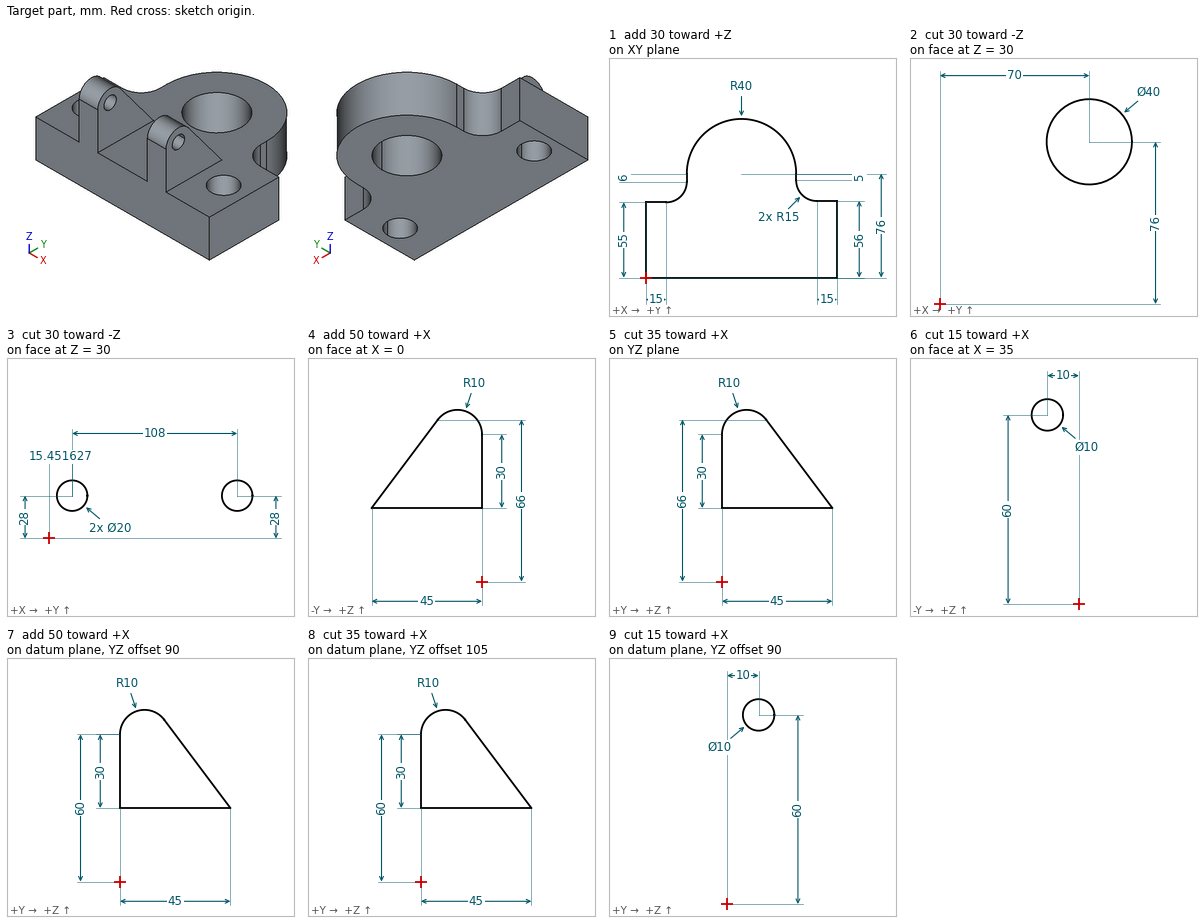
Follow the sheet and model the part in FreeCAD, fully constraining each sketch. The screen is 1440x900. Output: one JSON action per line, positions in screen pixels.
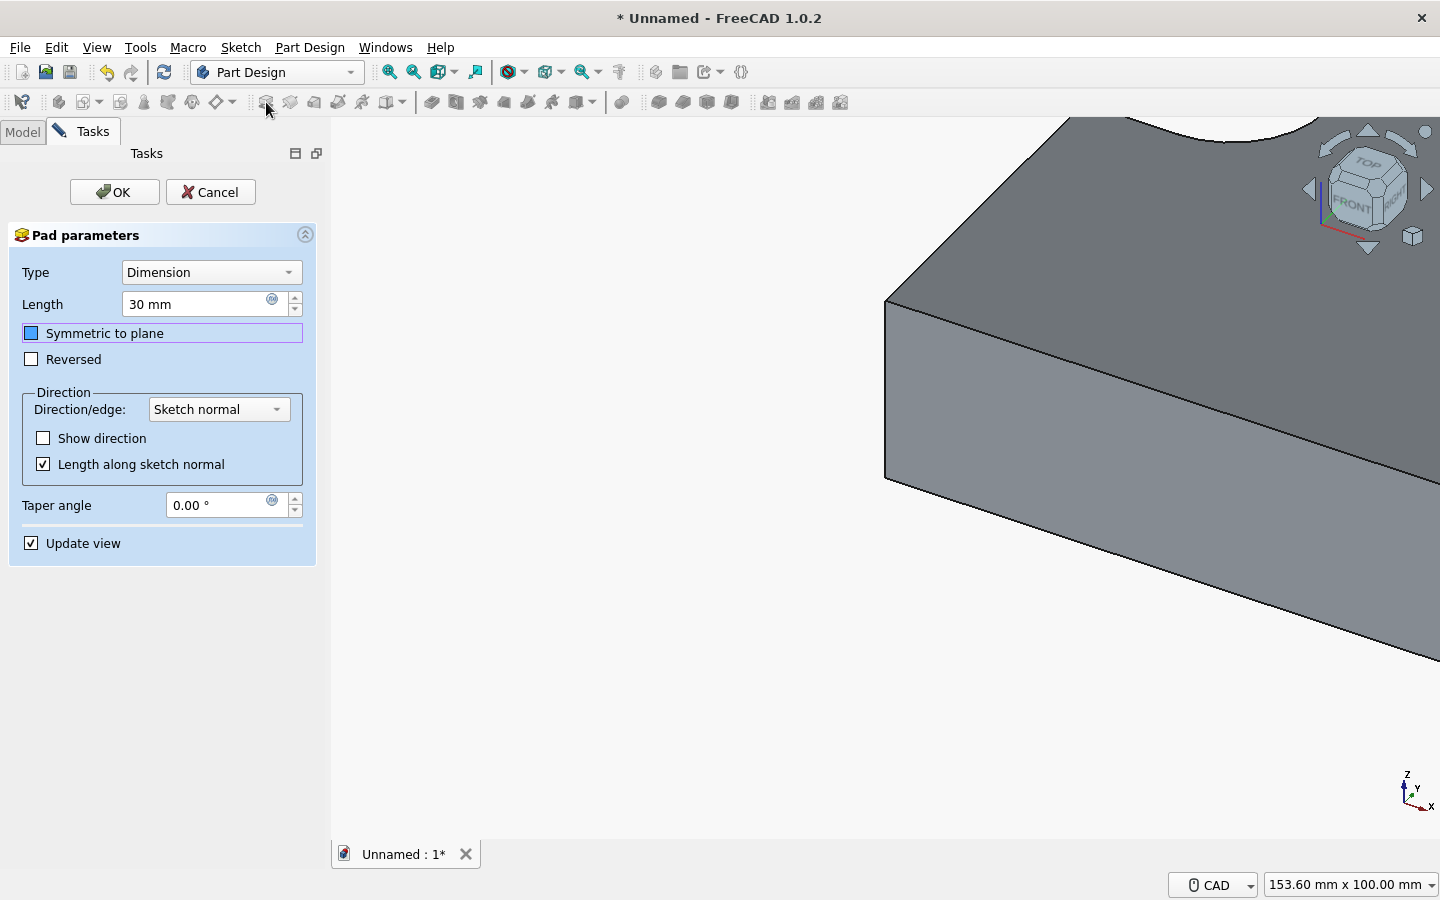
{"action": "left_click", "coordinate": [115, 192]}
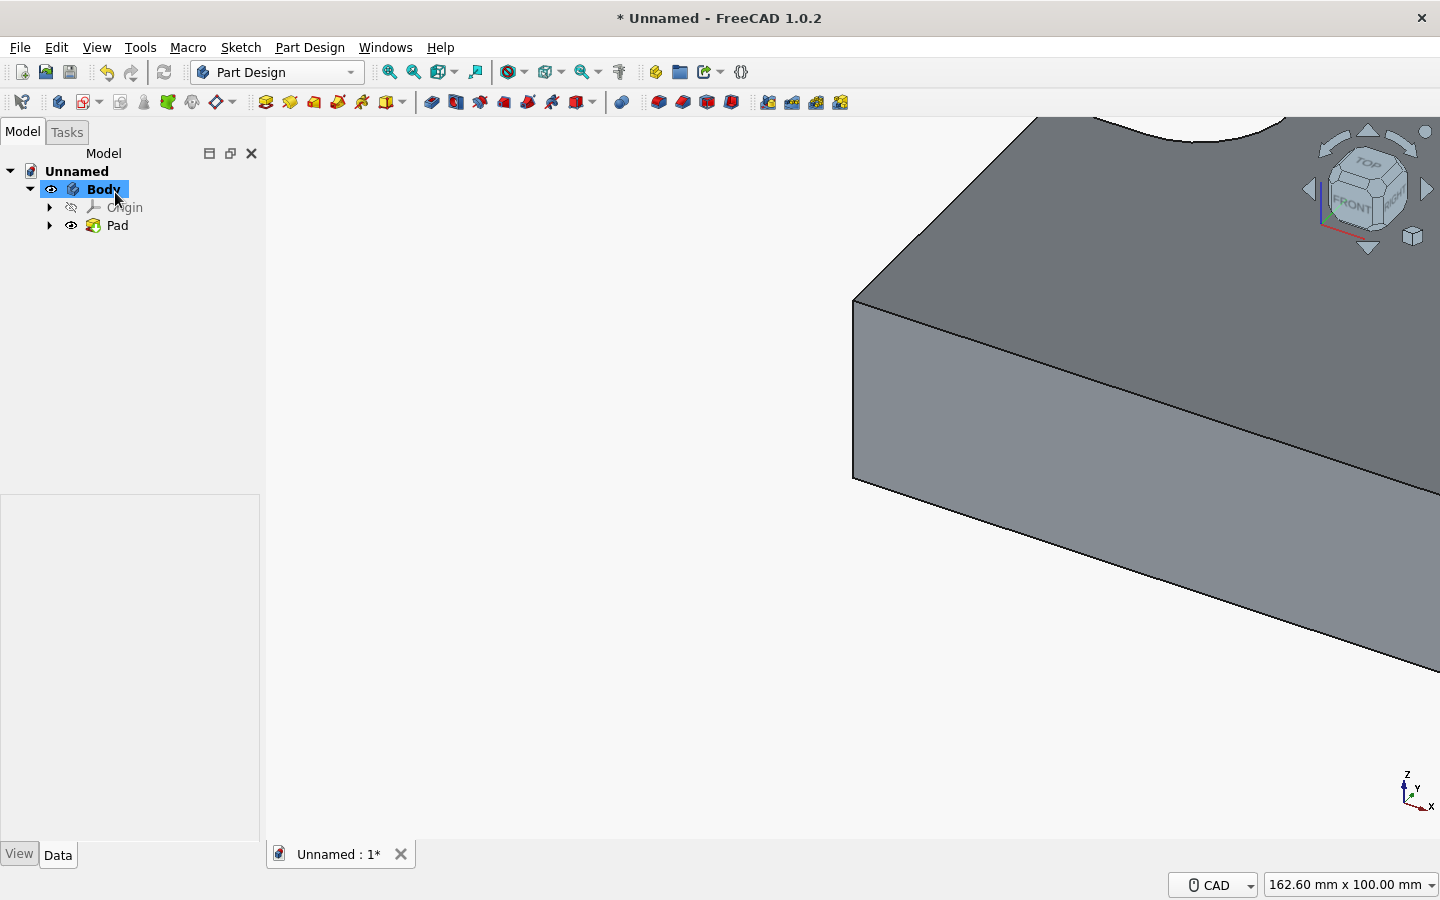
{"action": "key", "text": "v f"}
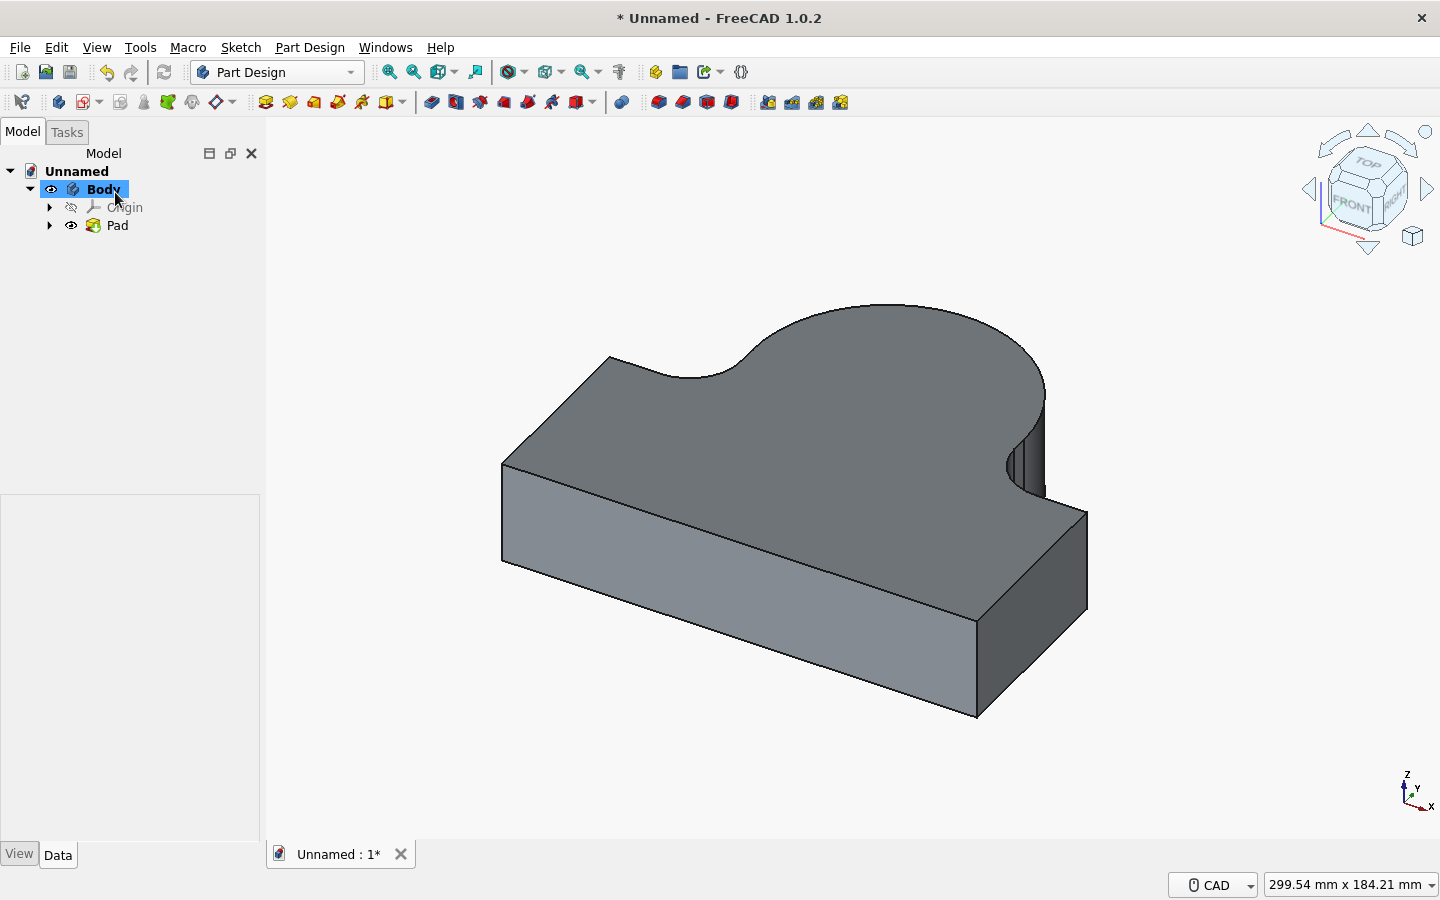
{"action": "left_click", "coordinate": [821, 461]}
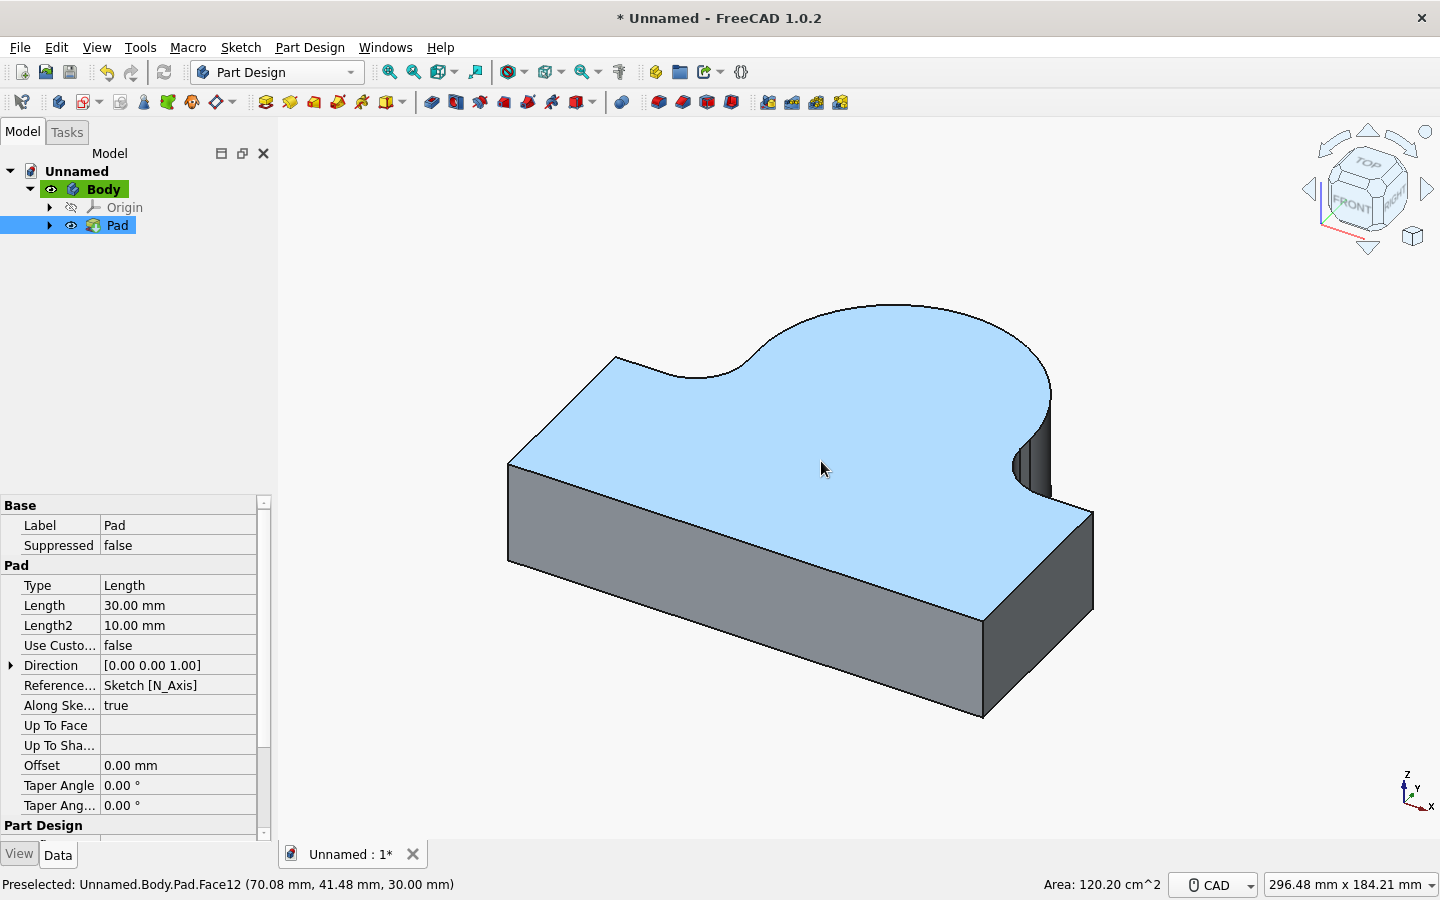
{"action": "left_click", "coordinate": [84, 102]}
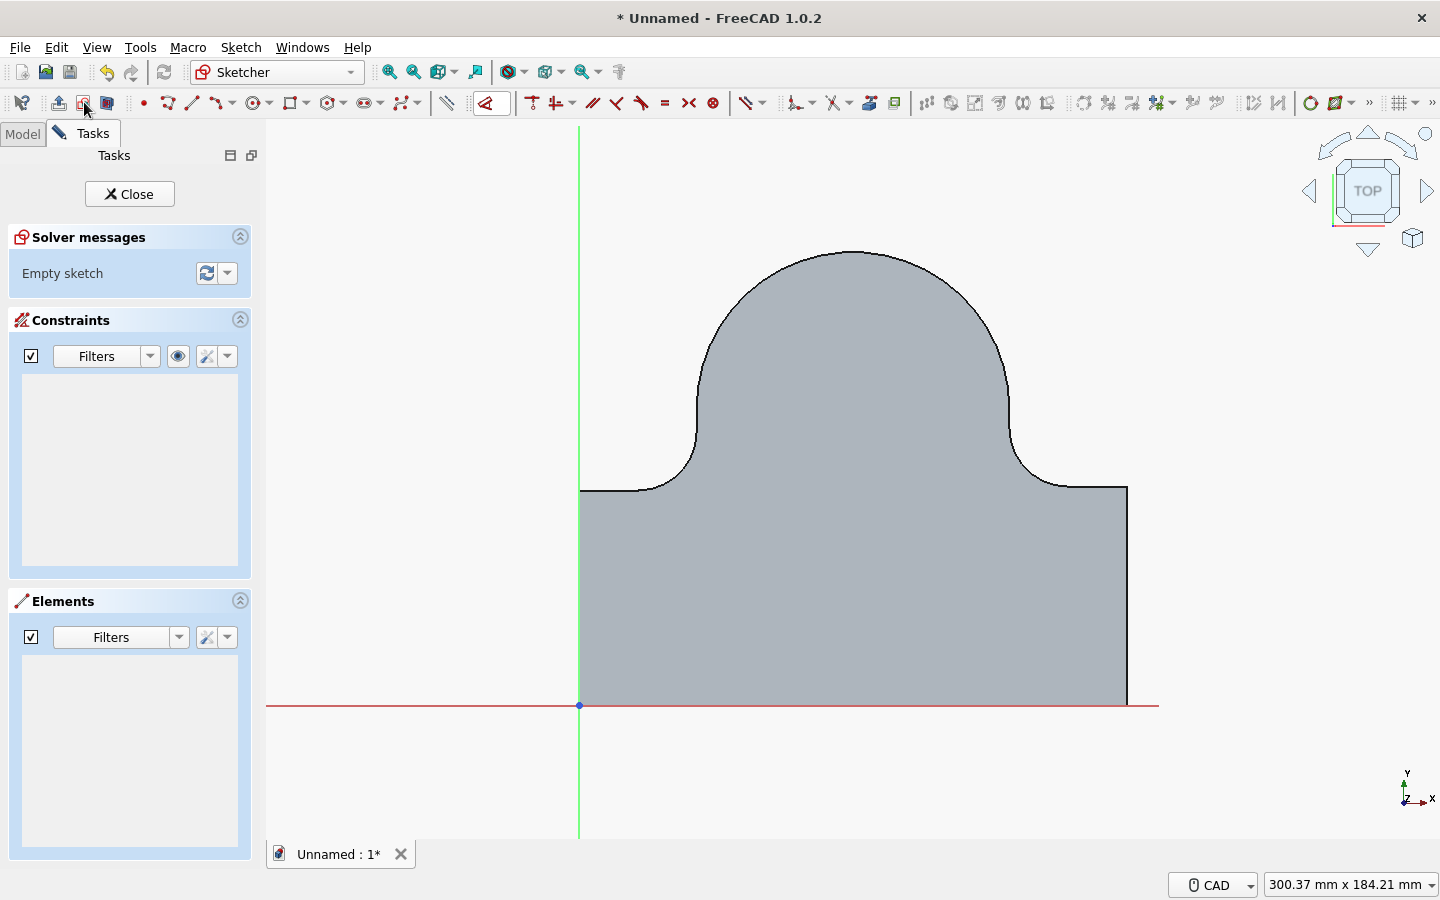
{"action": "key", "text": "g c"}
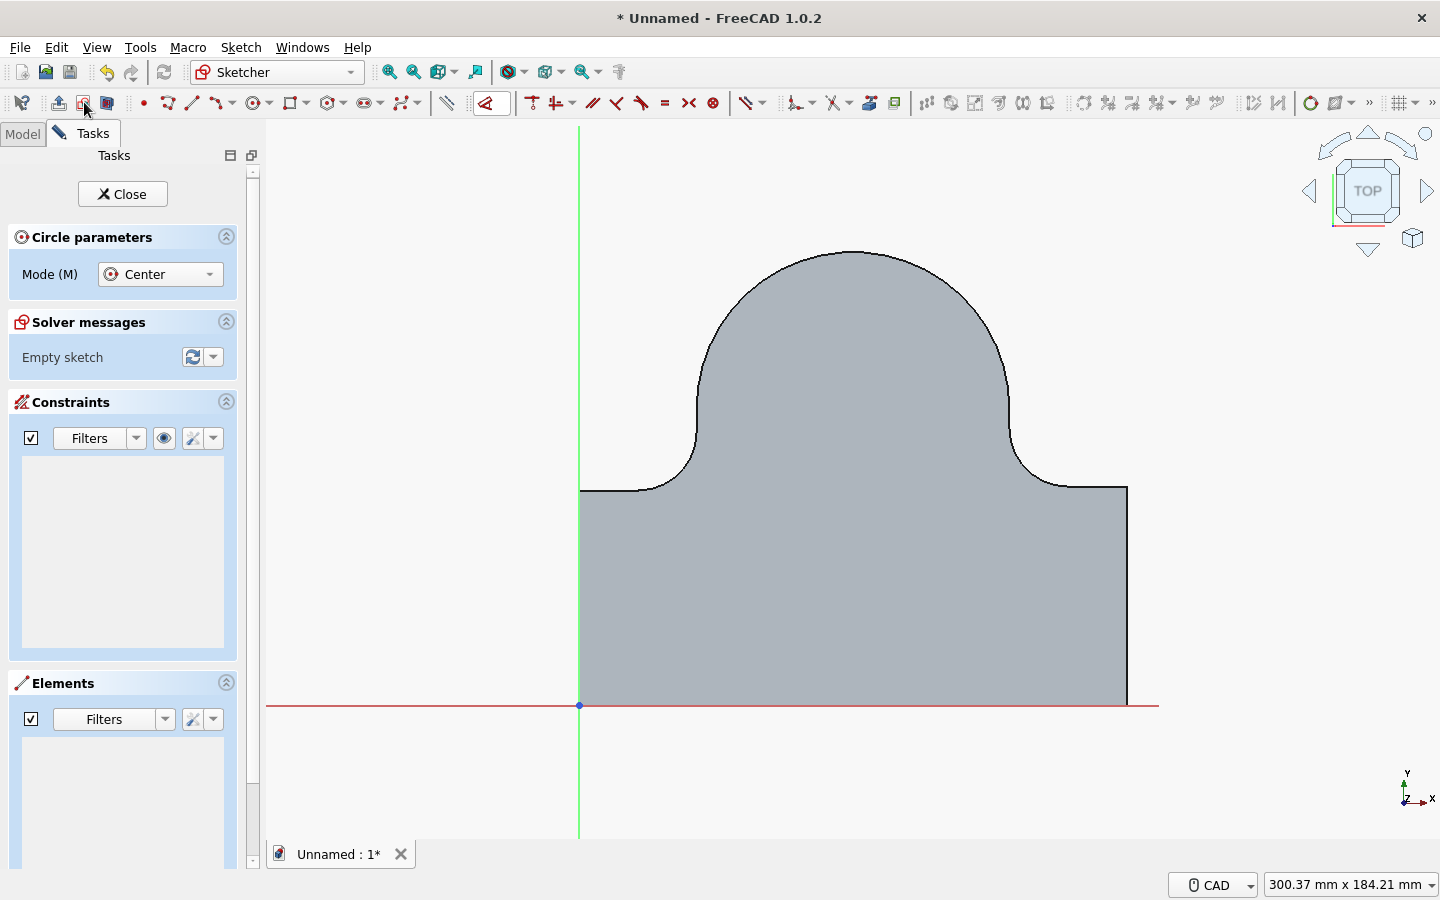
{"action": "left_click", "coordinate": [853, 408]}
{"action": "mouse_move", "coordinate": [908, 353]}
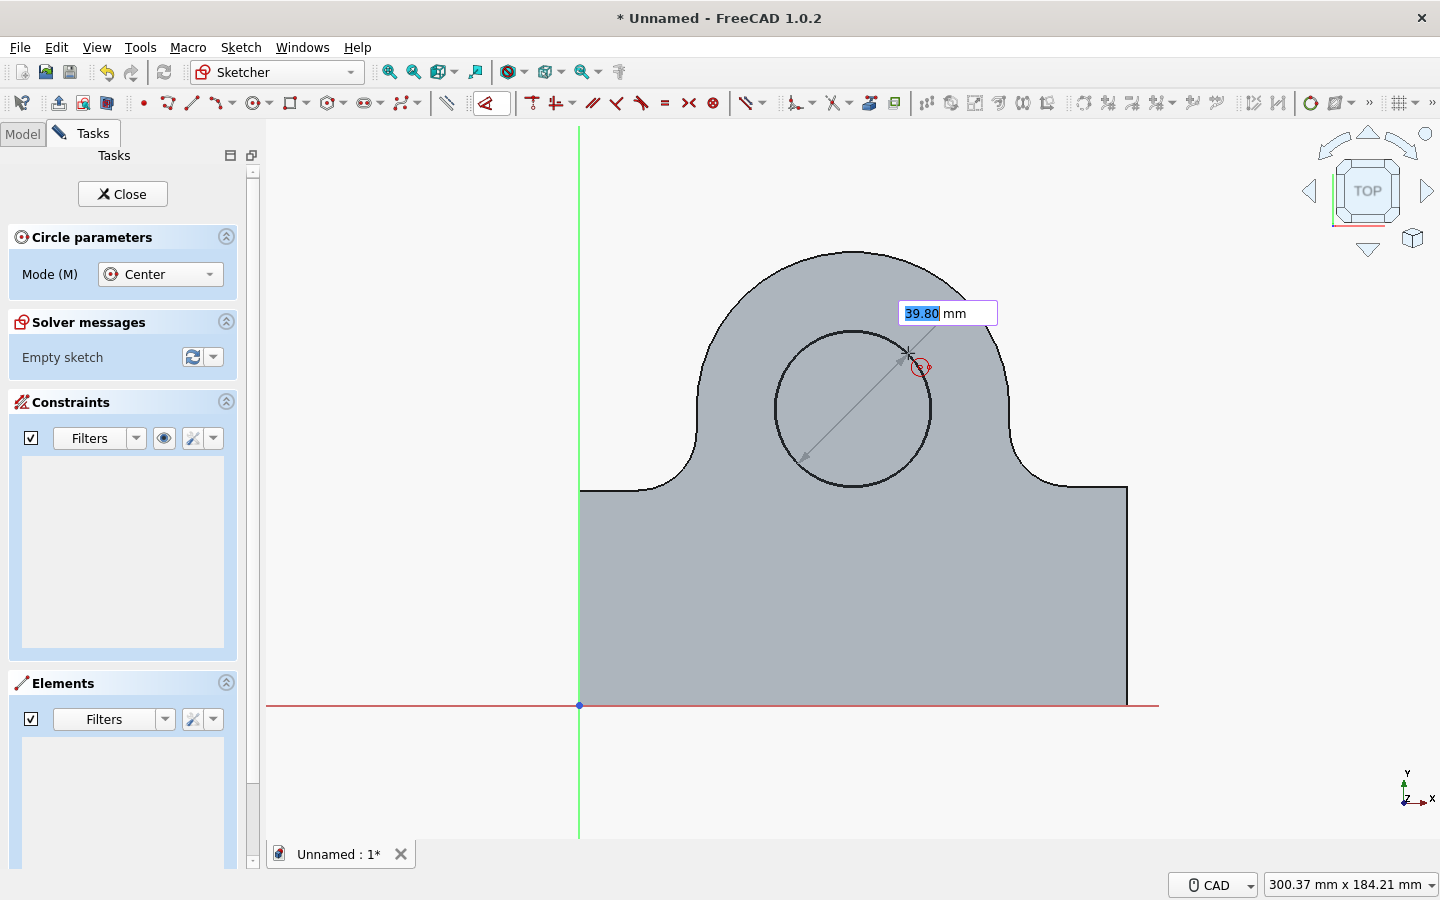
{"action": "type", "text": "40"}
{"action": "key", "text": "Return"}
{"action": "key", "text": "Escape"}